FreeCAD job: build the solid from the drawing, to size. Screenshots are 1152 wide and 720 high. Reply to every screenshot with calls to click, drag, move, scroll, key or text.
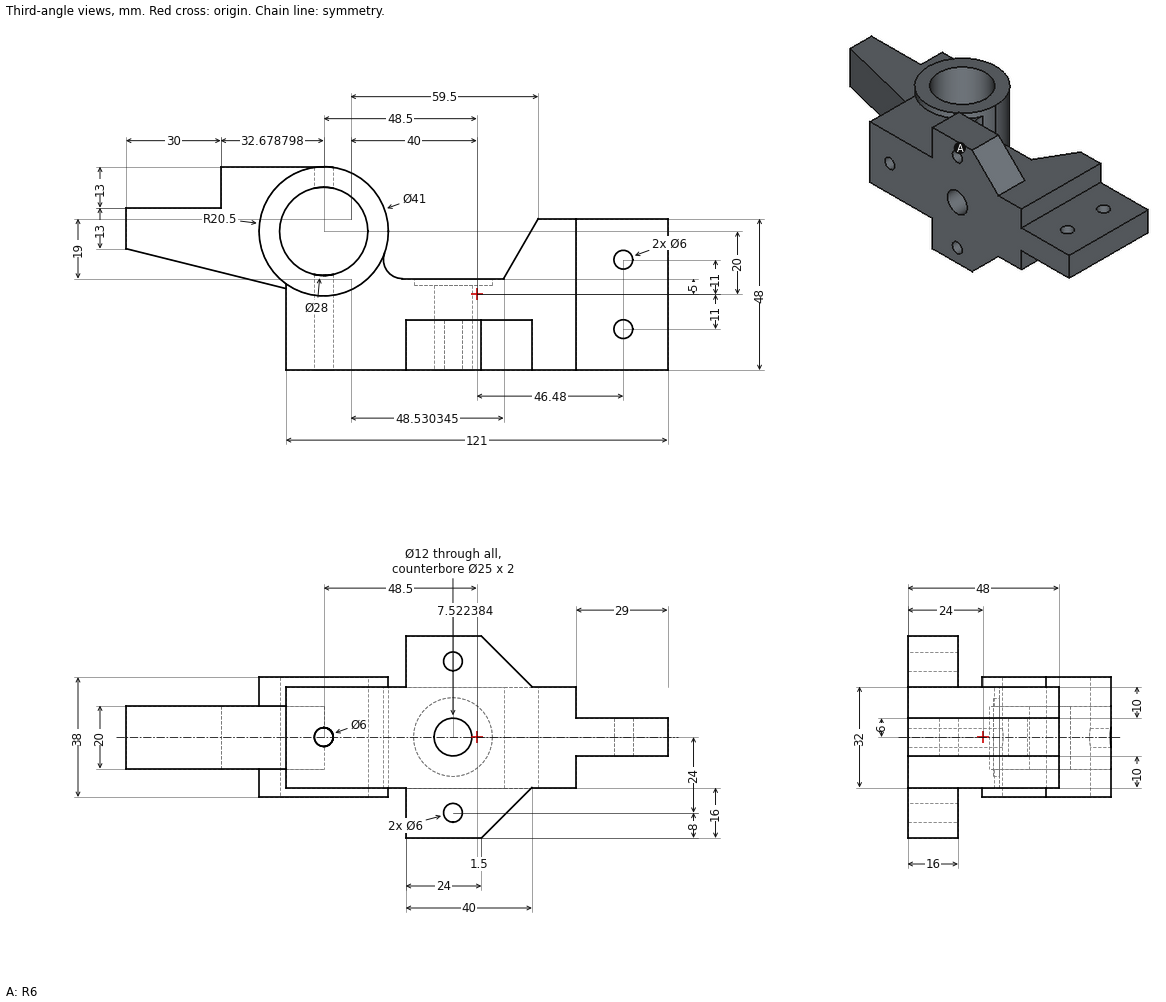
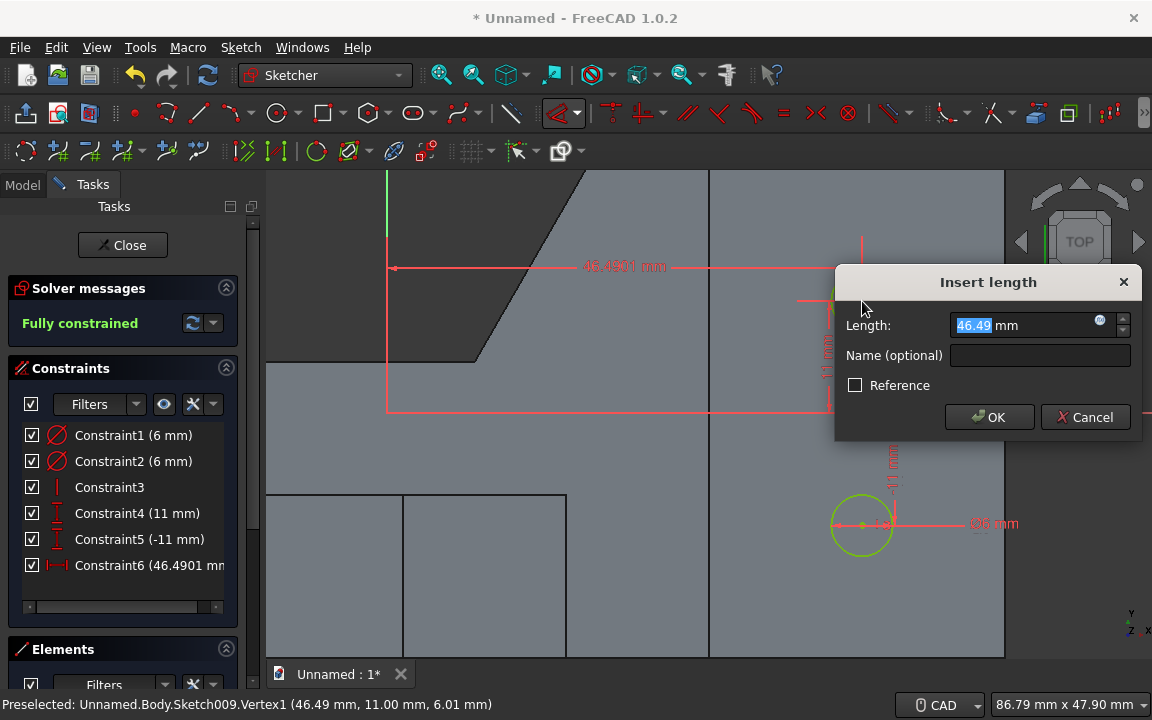
text(46.48)
key(Return)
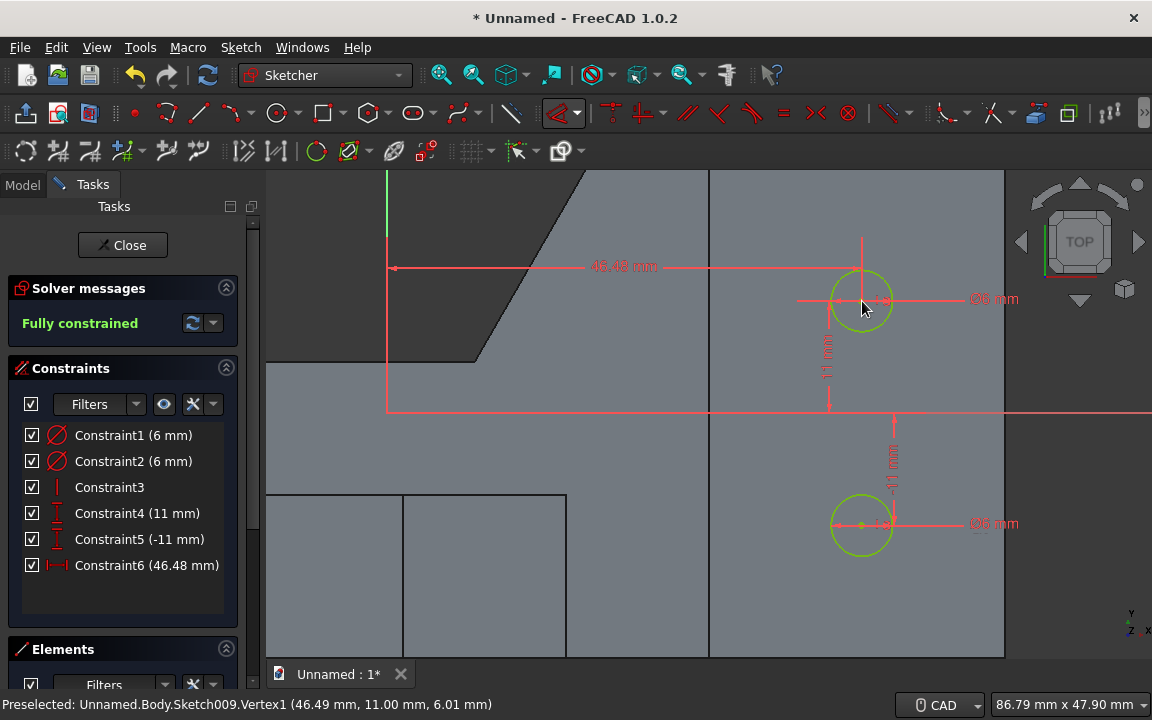
click(123, 245)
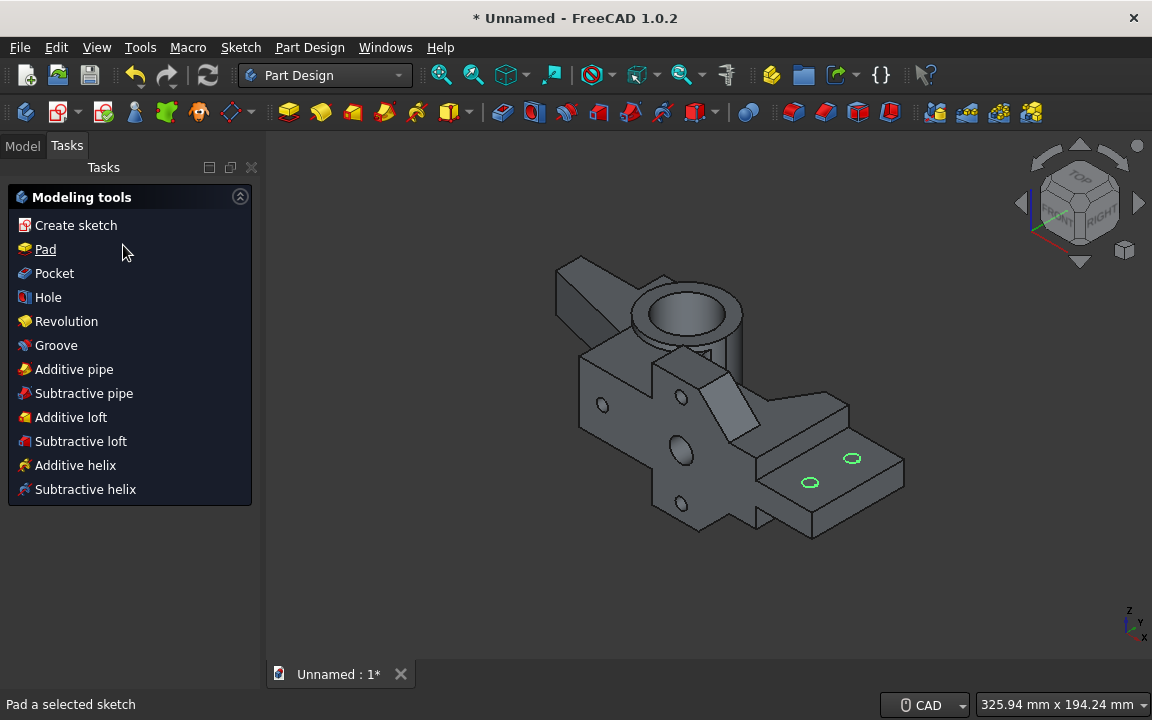
click(504, 112)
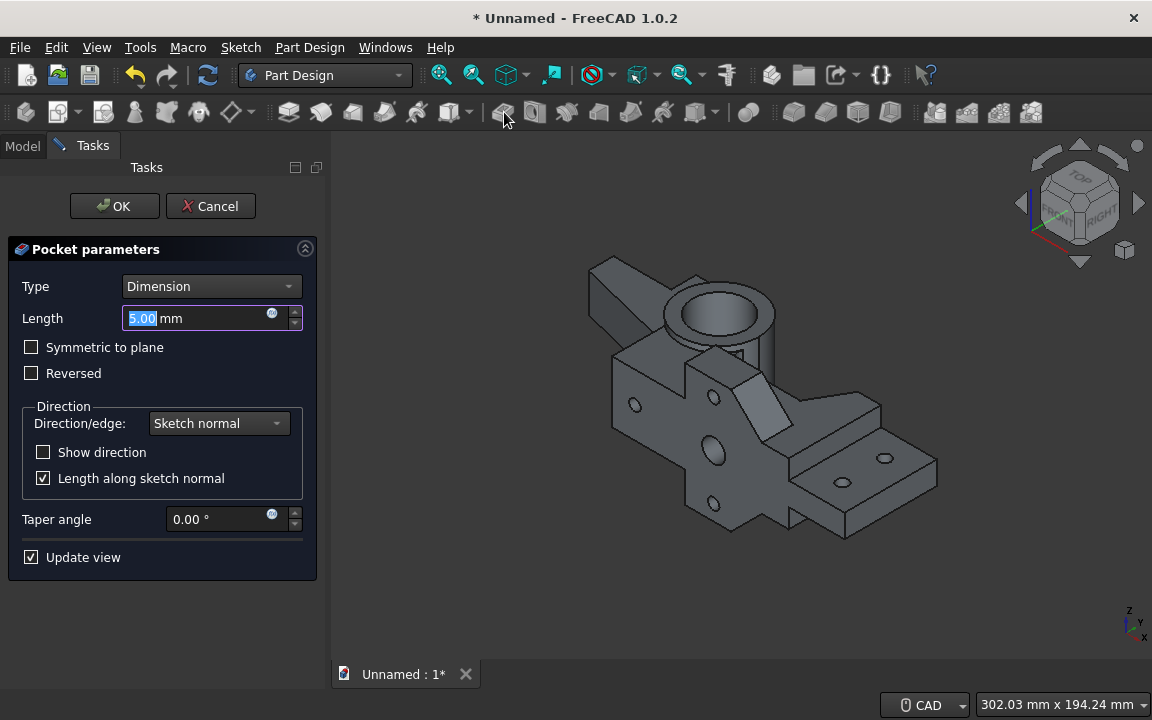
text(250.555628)
key(Tab)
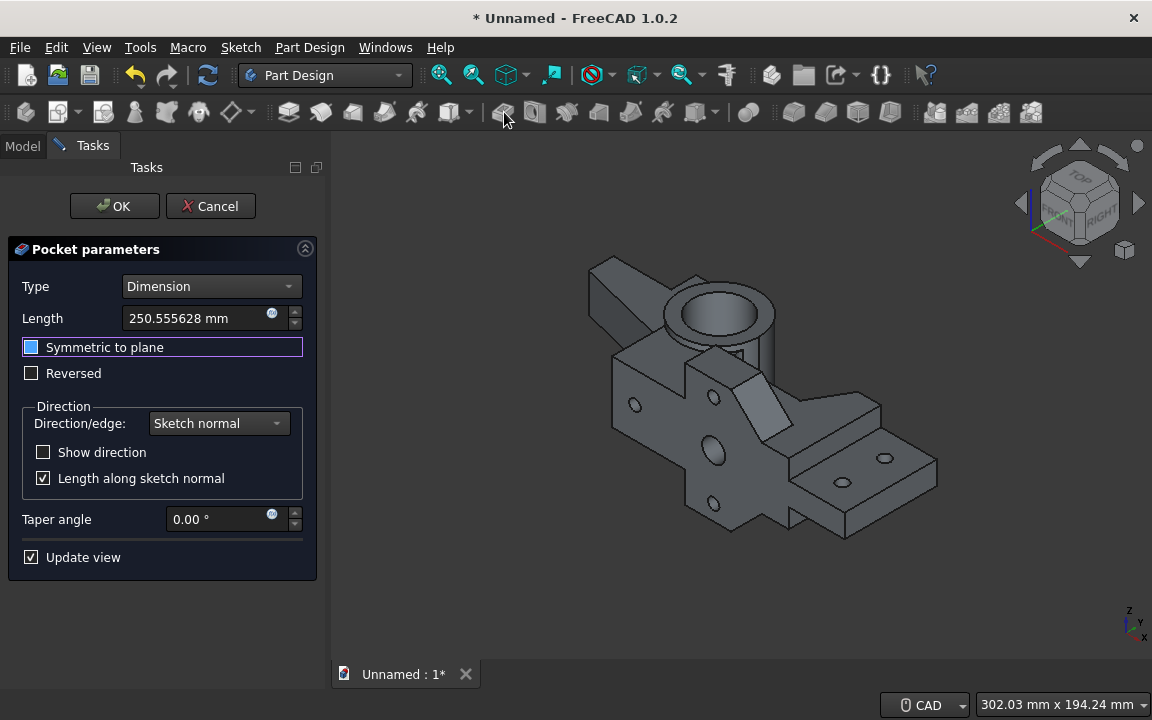
click(30, 347)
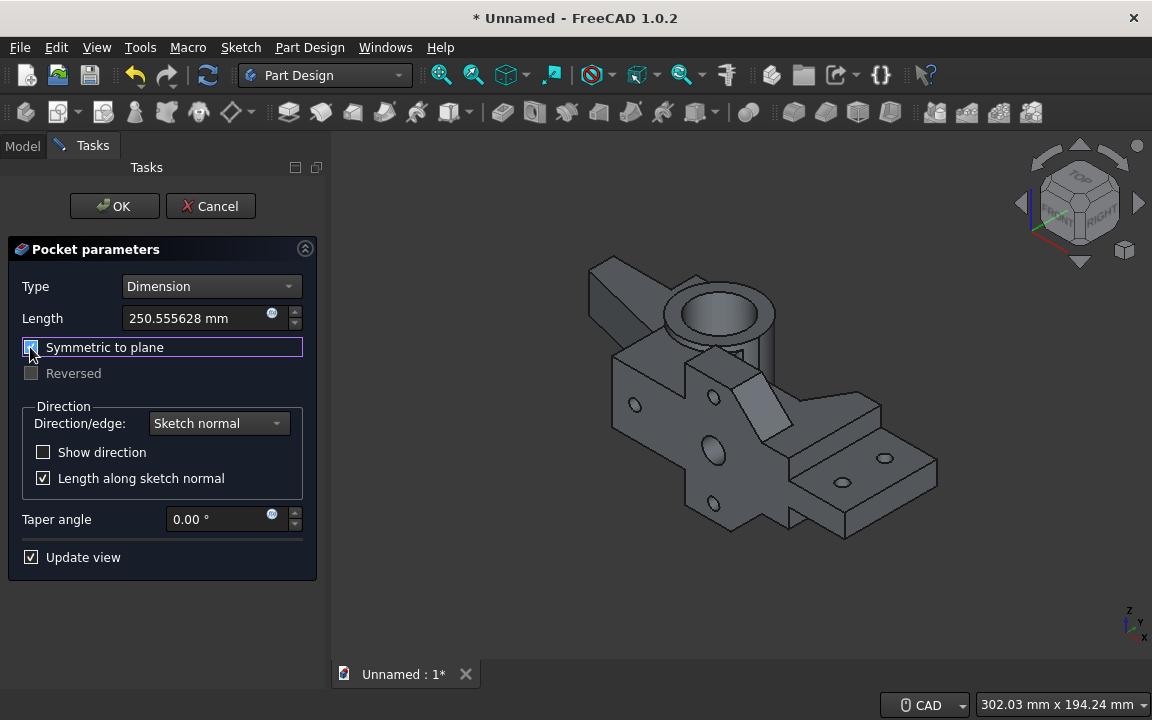
click(115, 206)